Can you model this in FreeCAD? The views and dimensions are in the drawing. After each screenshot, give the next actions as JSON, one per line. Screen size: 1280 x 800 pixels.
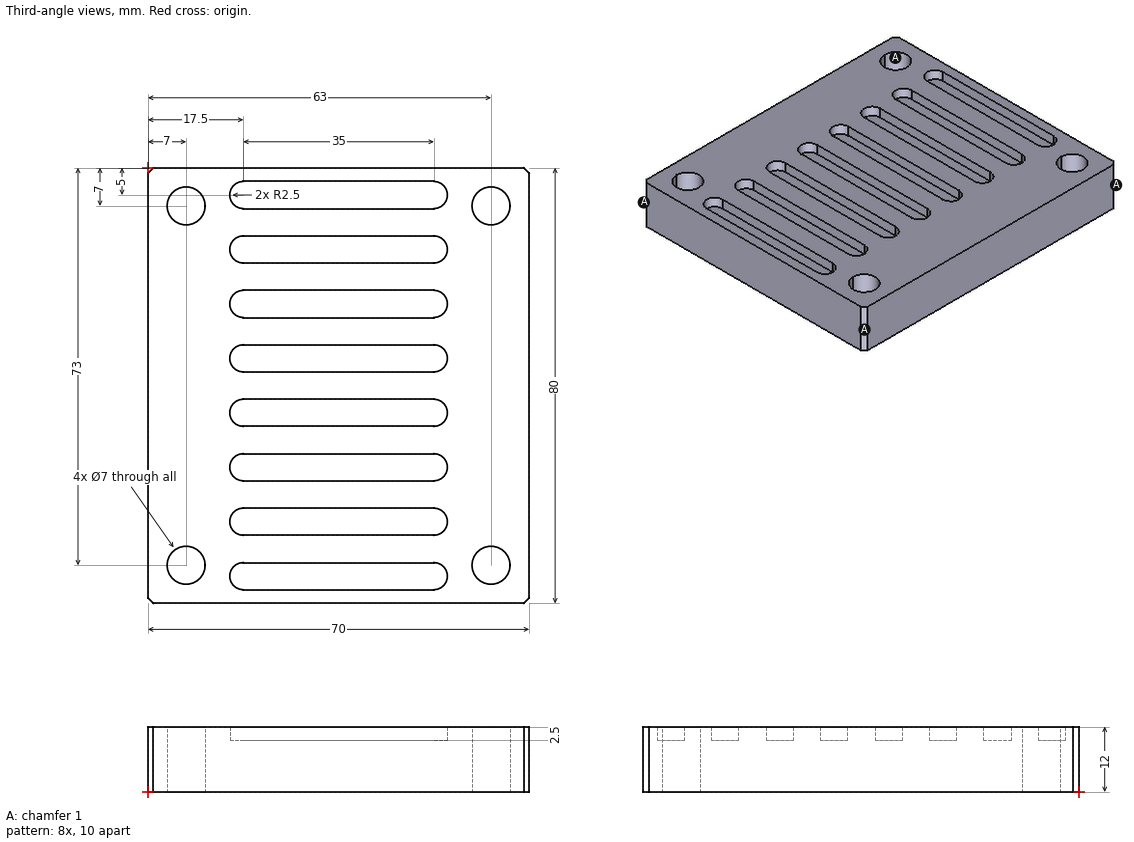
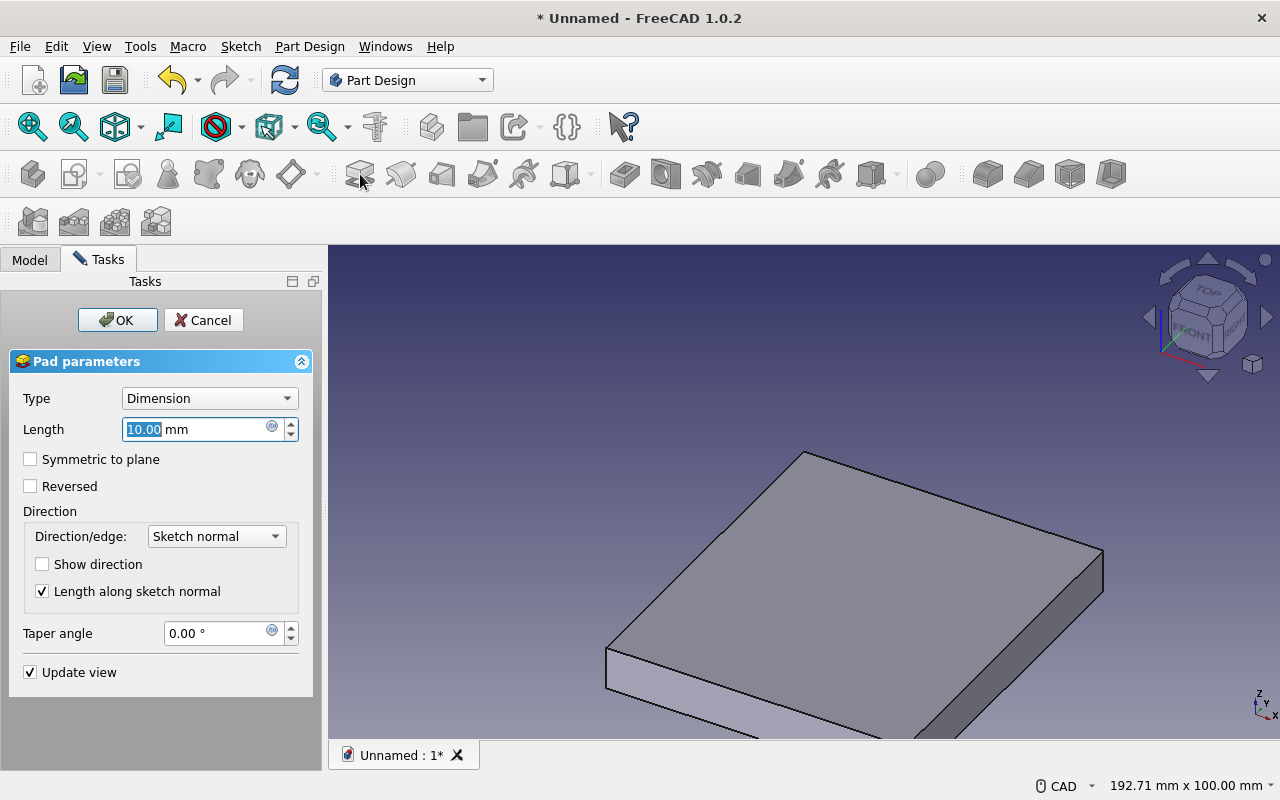
{"action": "type", "text": "12"}
{"action": "key", "text": "Tab"}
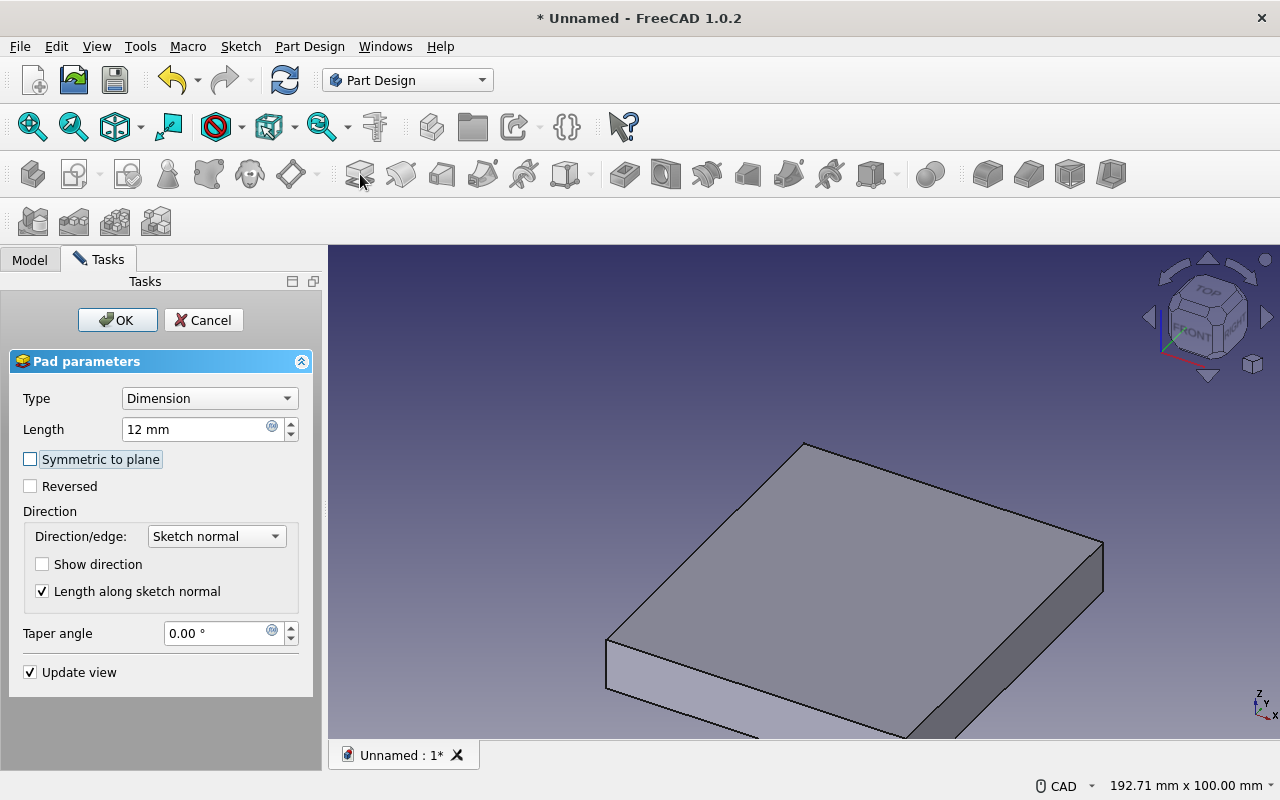
{"action": "left_click", "coordinate": [118, 320]}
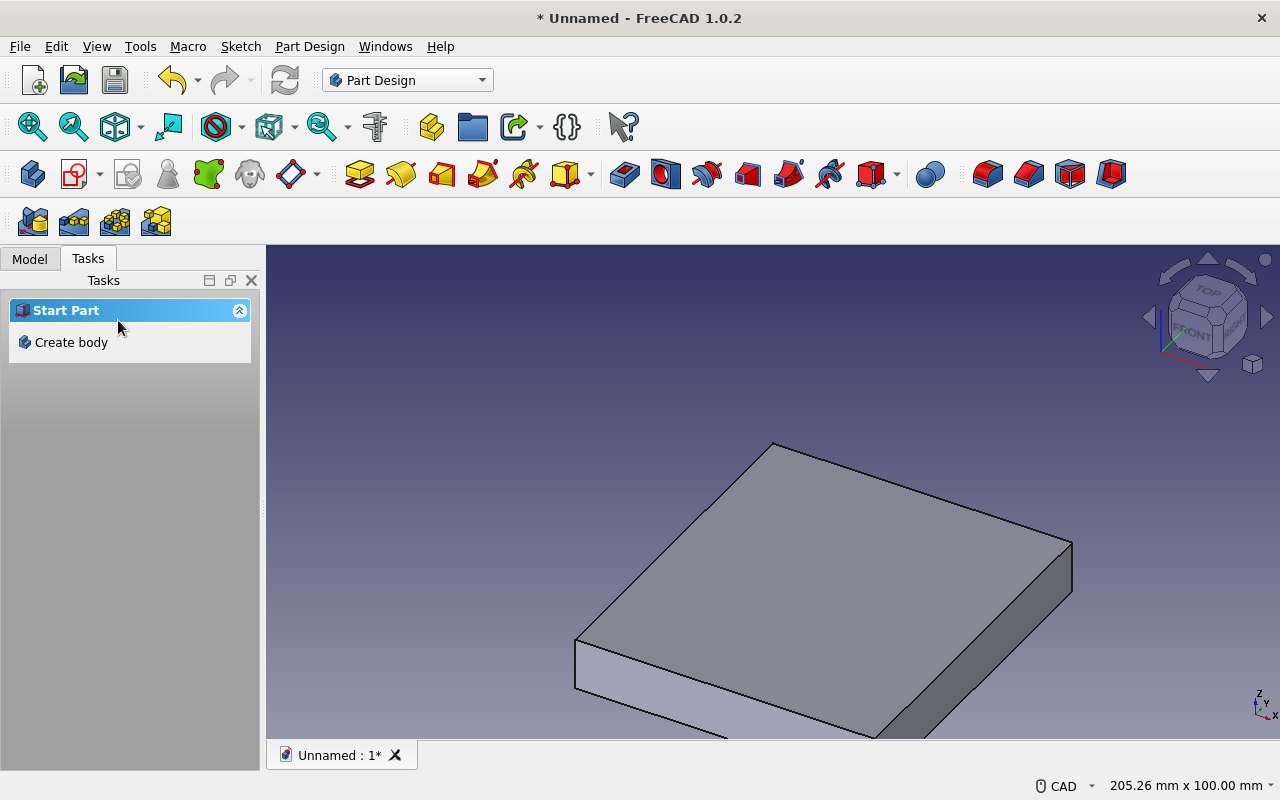
{"action": "key", "text": "v f"}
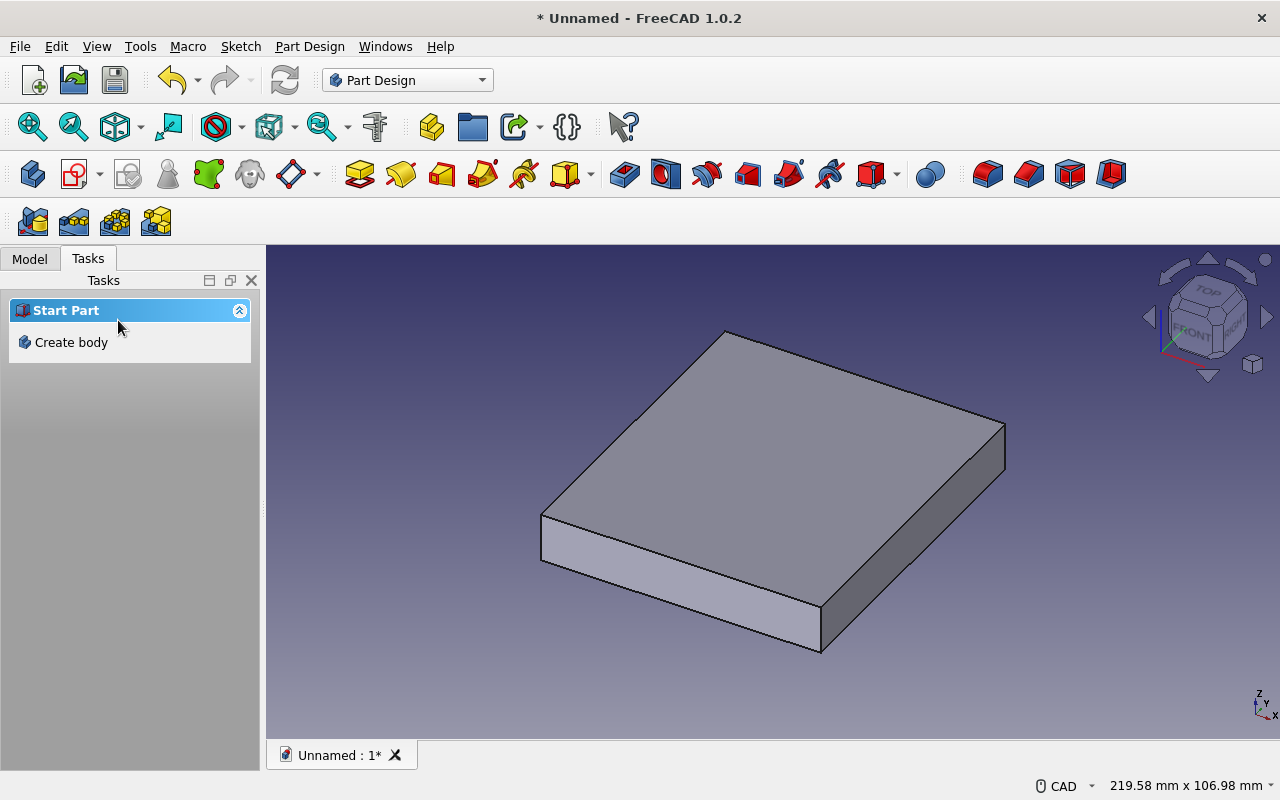
{"action": "left_click", "coordinate": [821, 629]}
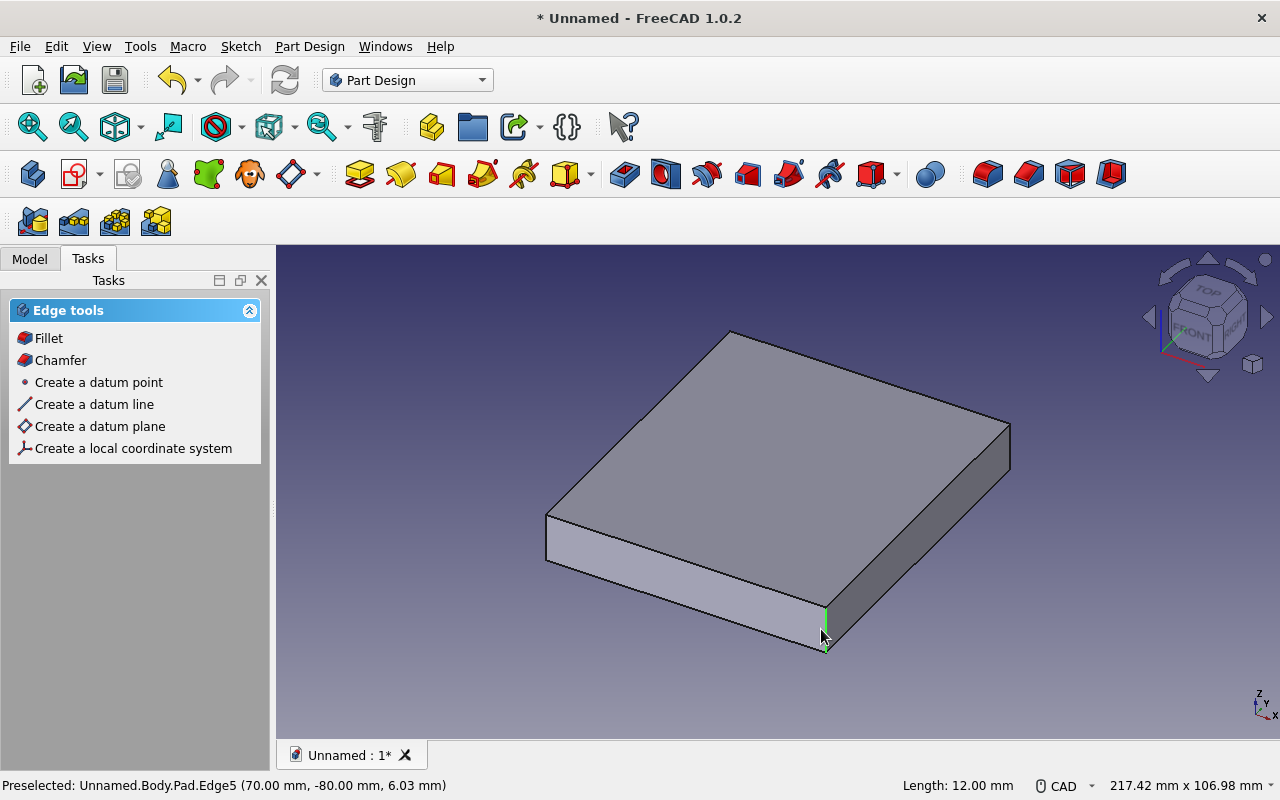
{"action": "key", "text": "0"}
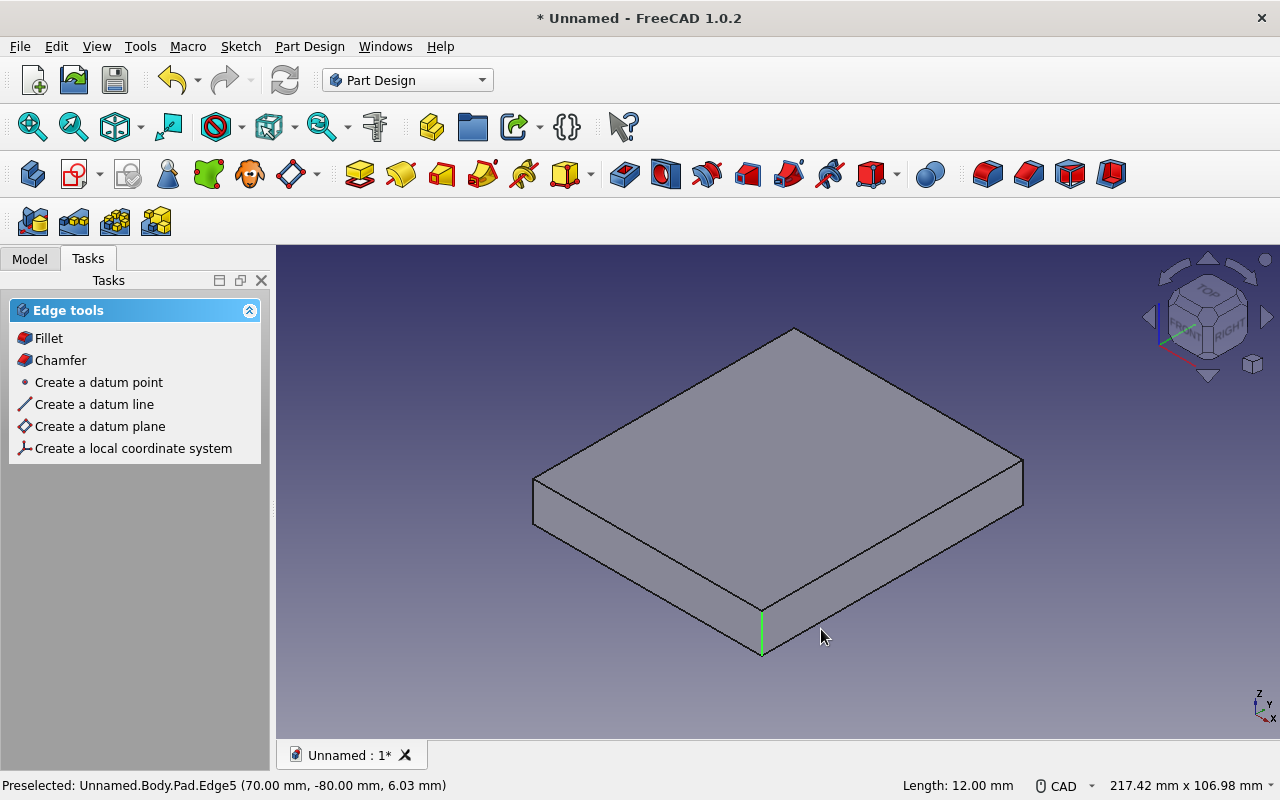
{"action": "key", "text": "2"}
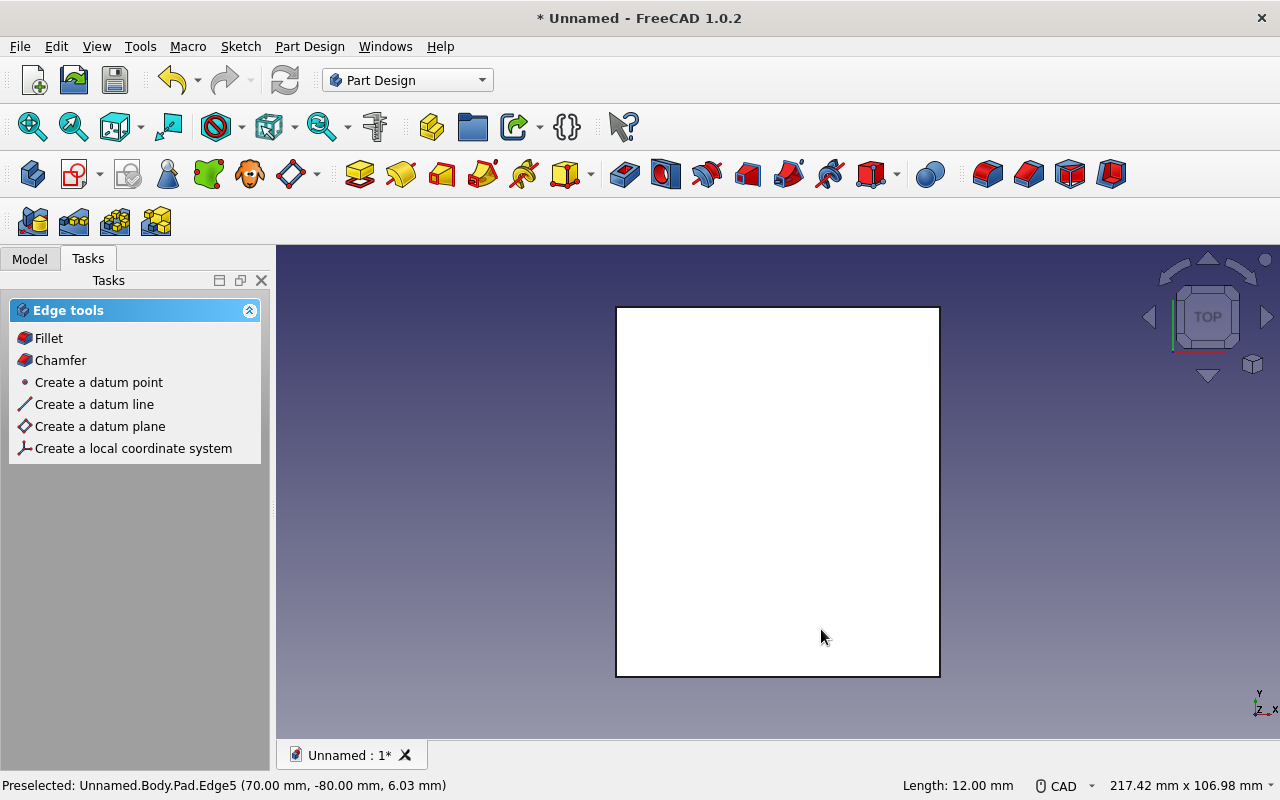
{"action": "key", "text": "1"}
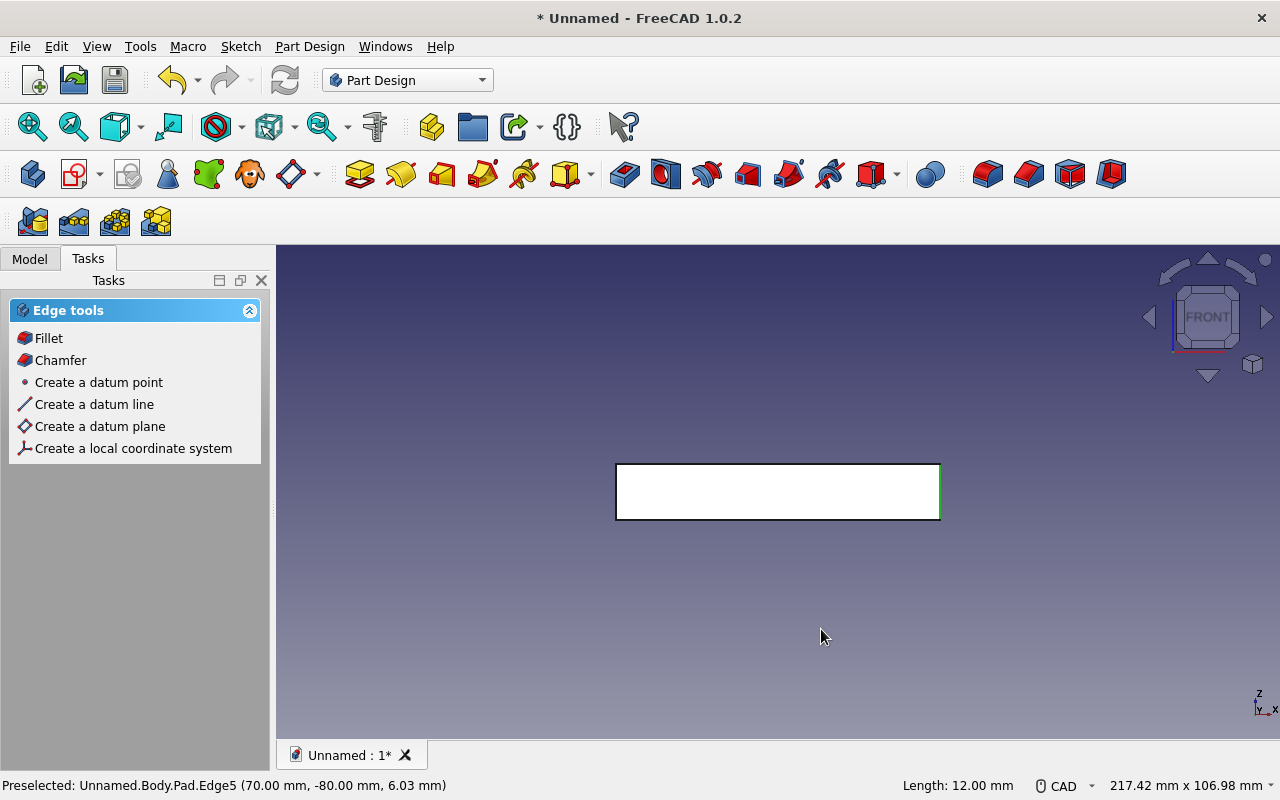
{"action": "key", "text": "v f"}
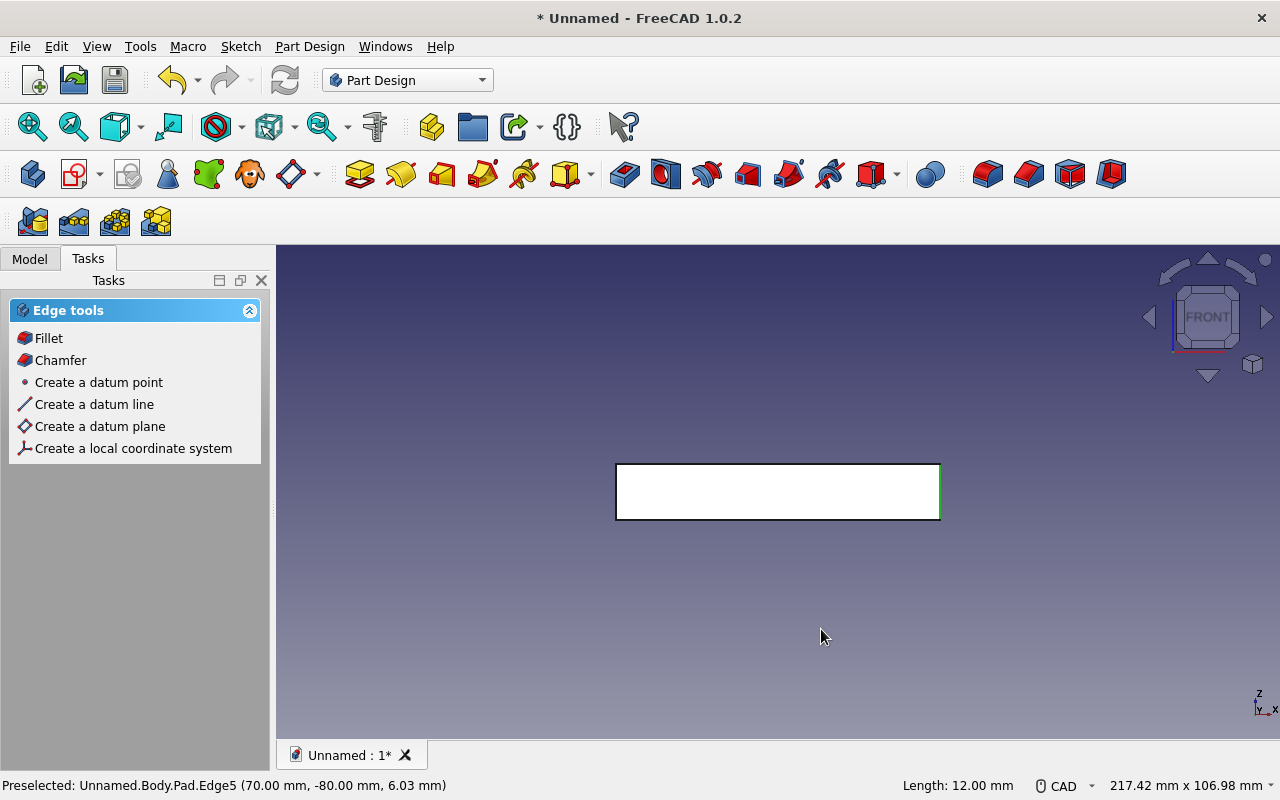
{"action": "left_click", "coordinate": [616, 491], "text": "ctrl"}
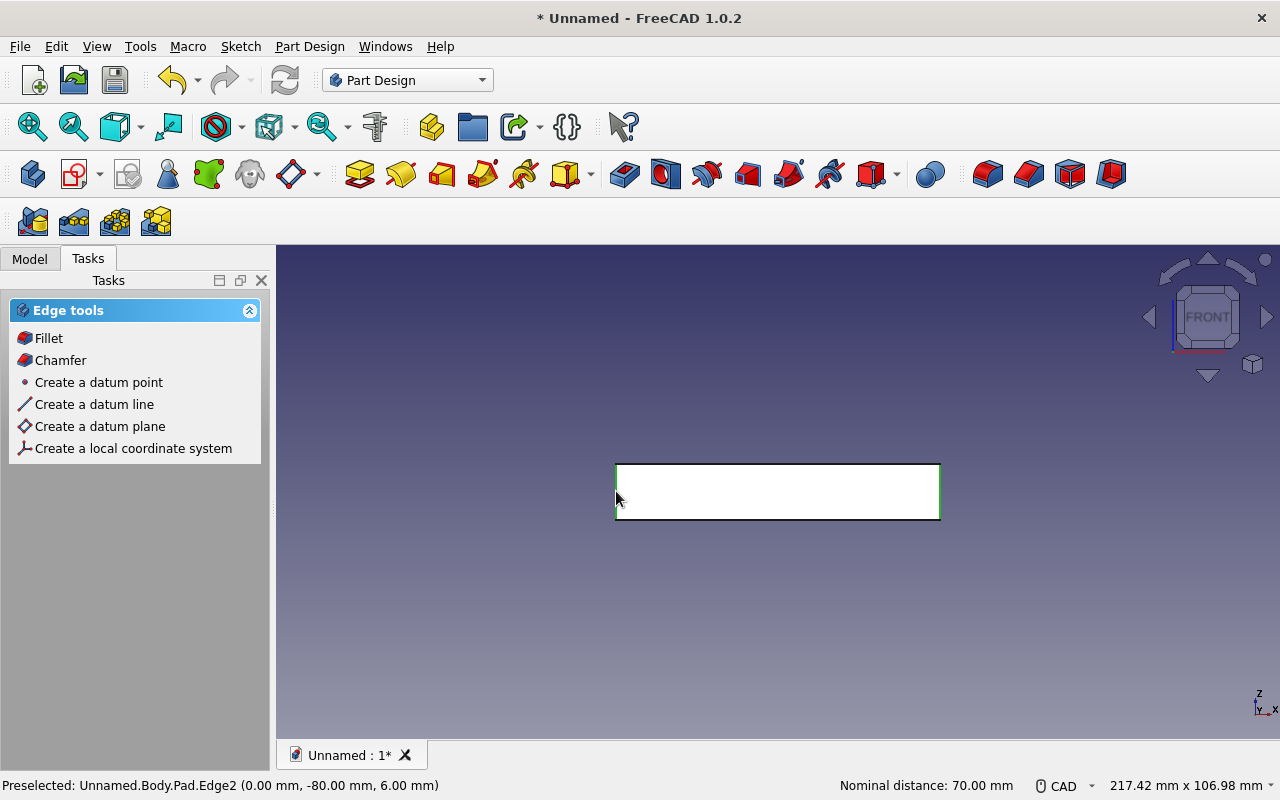
{"action": "key", "text": "3"}